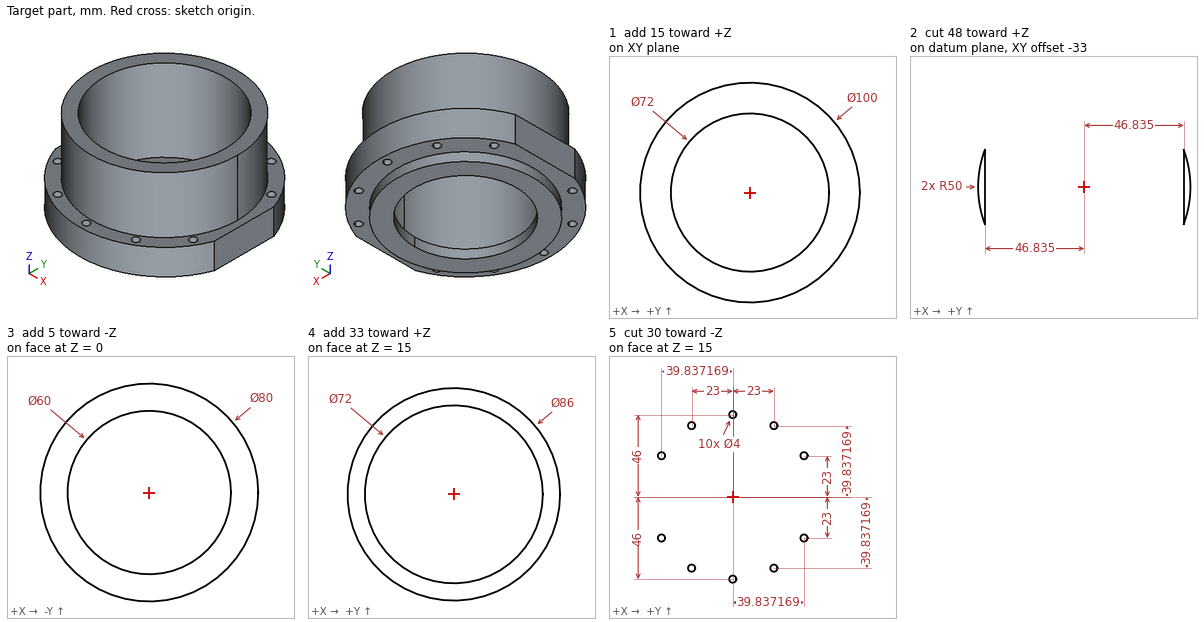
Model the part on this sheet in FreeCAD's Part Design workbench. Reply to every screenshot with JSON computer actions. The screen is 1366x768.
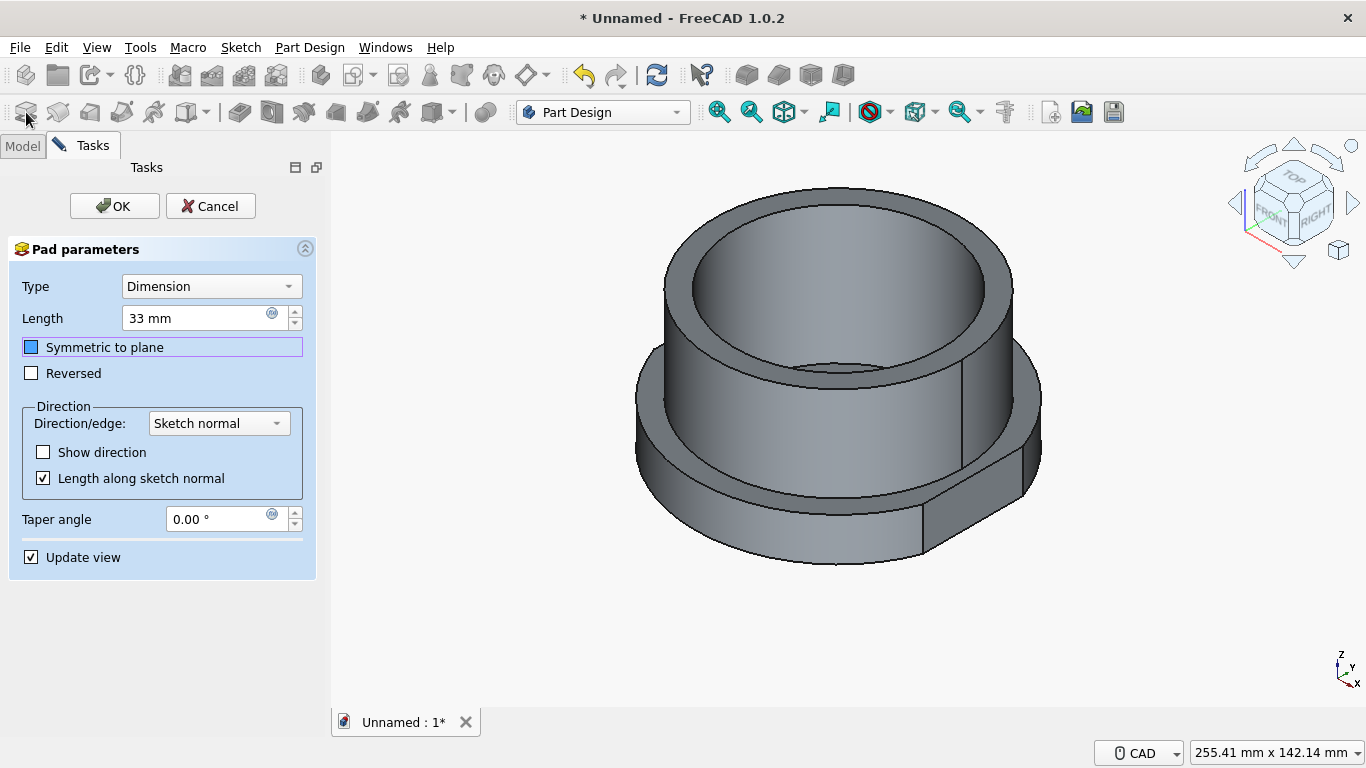
{"action": "left_click", "coordinate": [115, 206]}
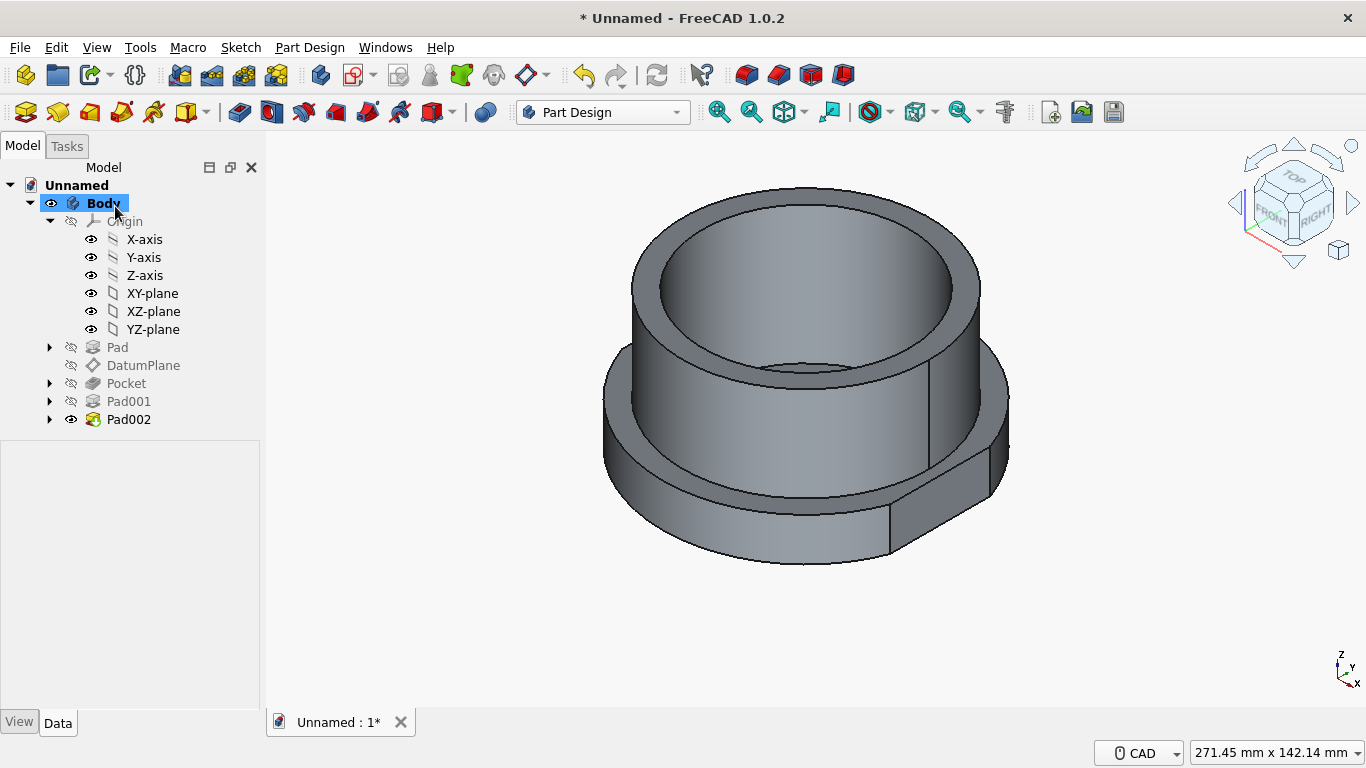
{"action": "left_click", "coordinate": [720, 112]}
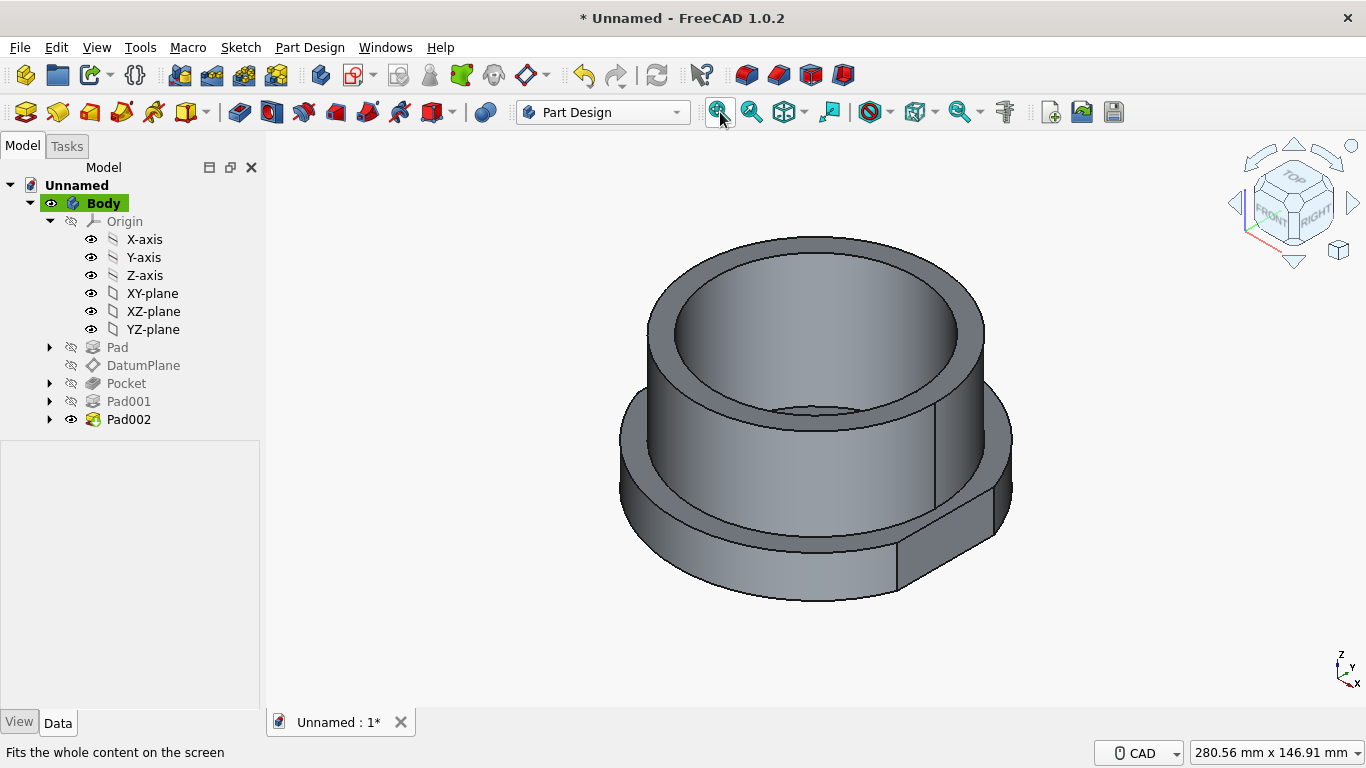
{"action": "left_click", "coordinate": [660, 486]}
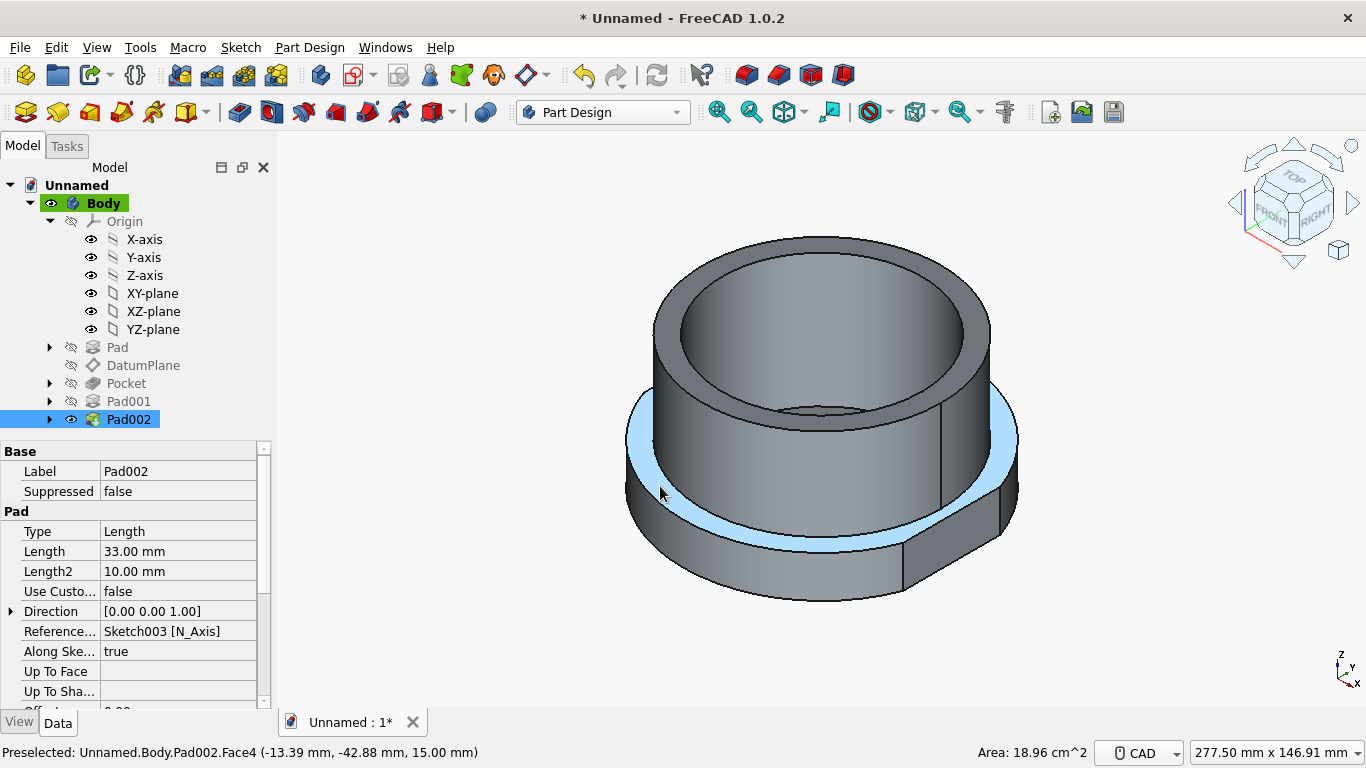
{"action": "left_click", "coordinate": [354, 76]}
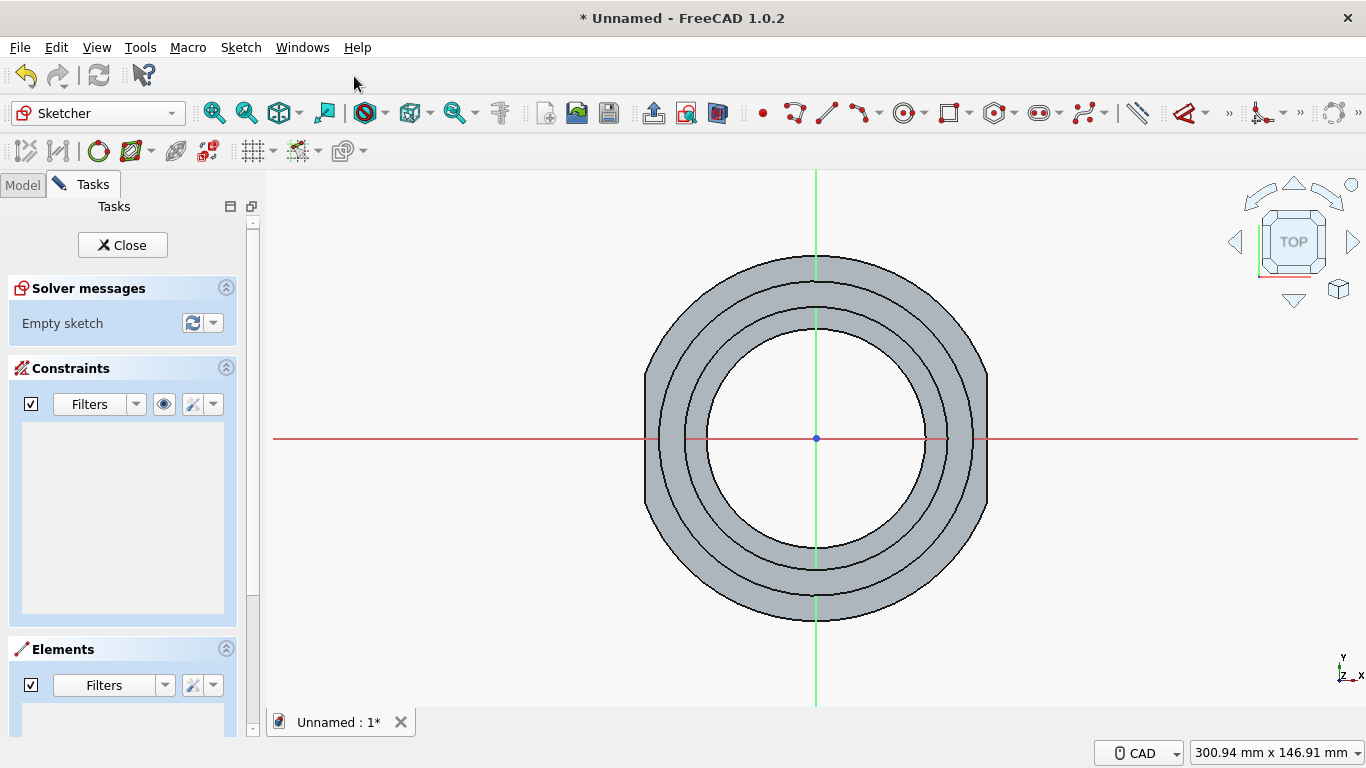
{"action": "left_click", "coordinate": [718, 114]}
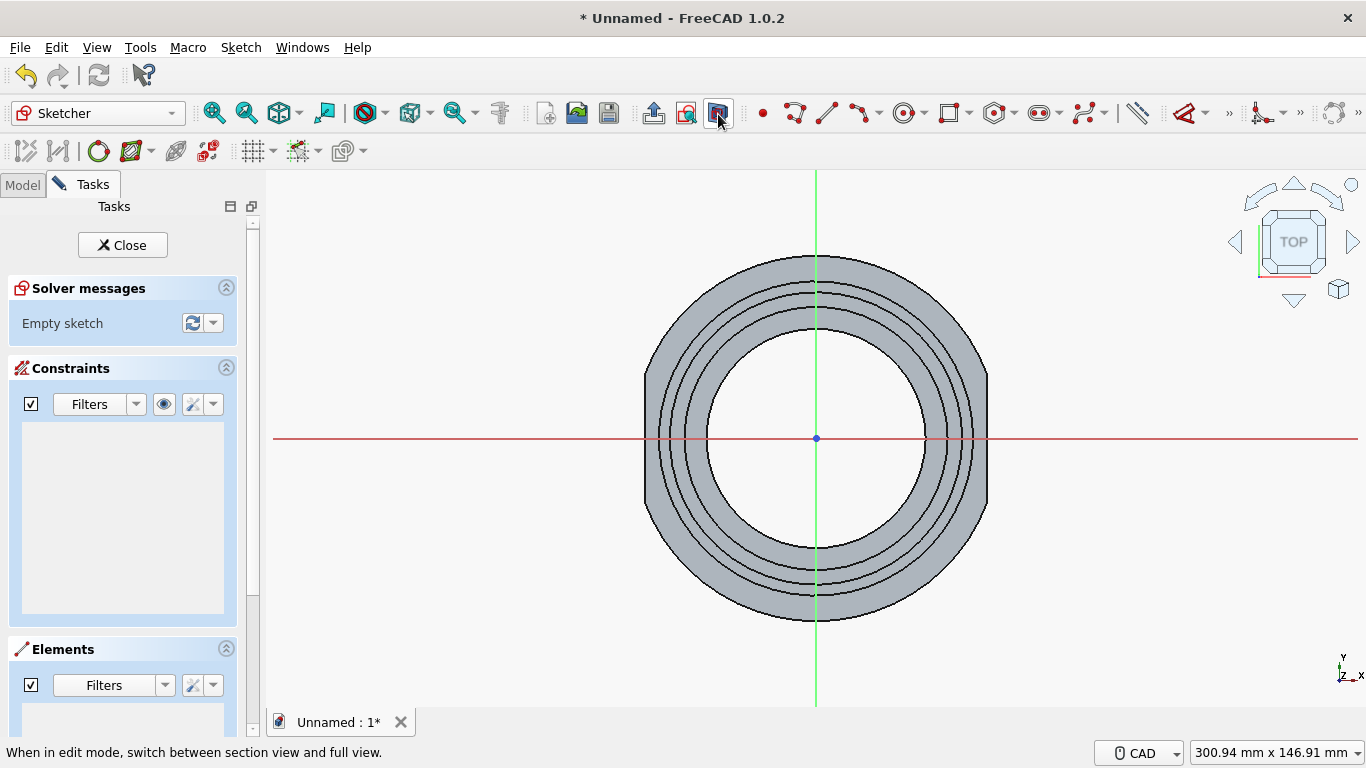
{"action": "left_click", "coordinate": [904, 114]}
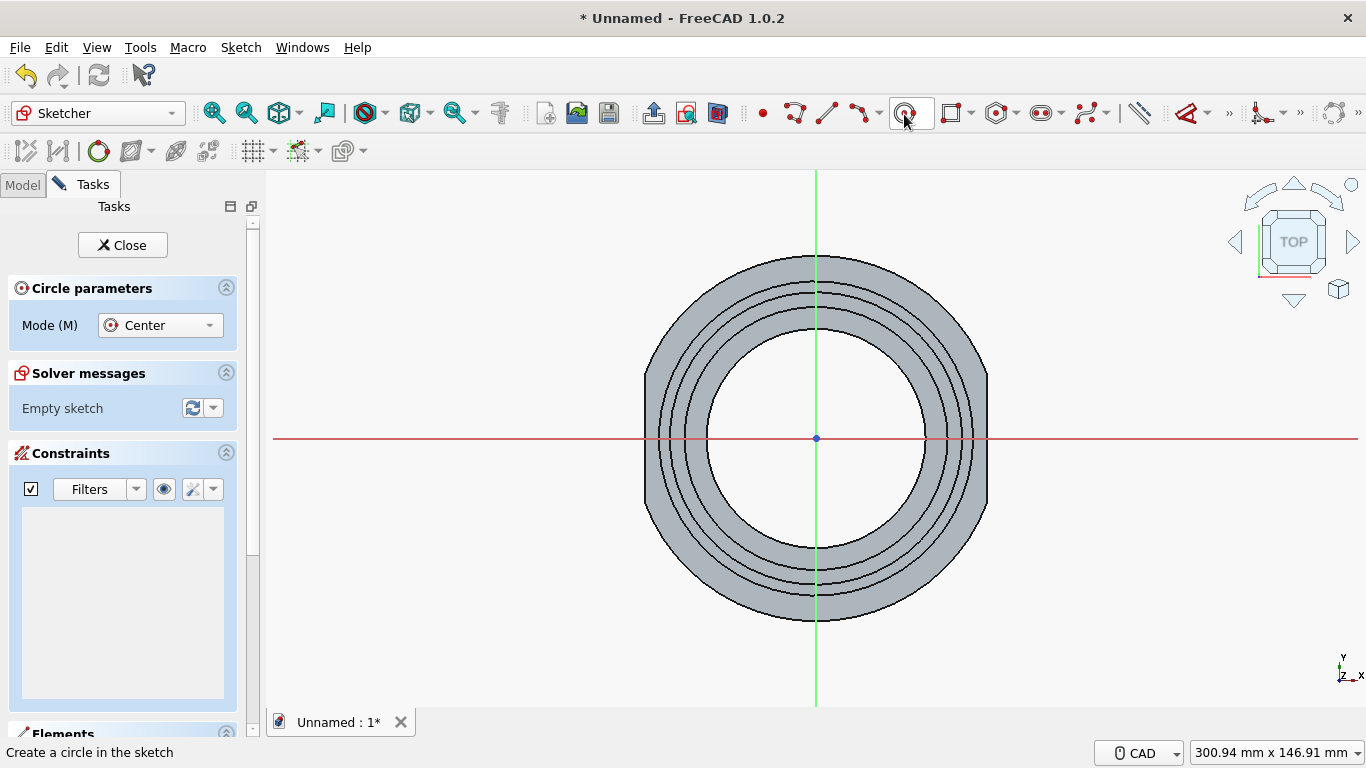
{"action": "scroll", "coordinate": [816, 270], "scroll_direction": "up", "scroll_amount": 6}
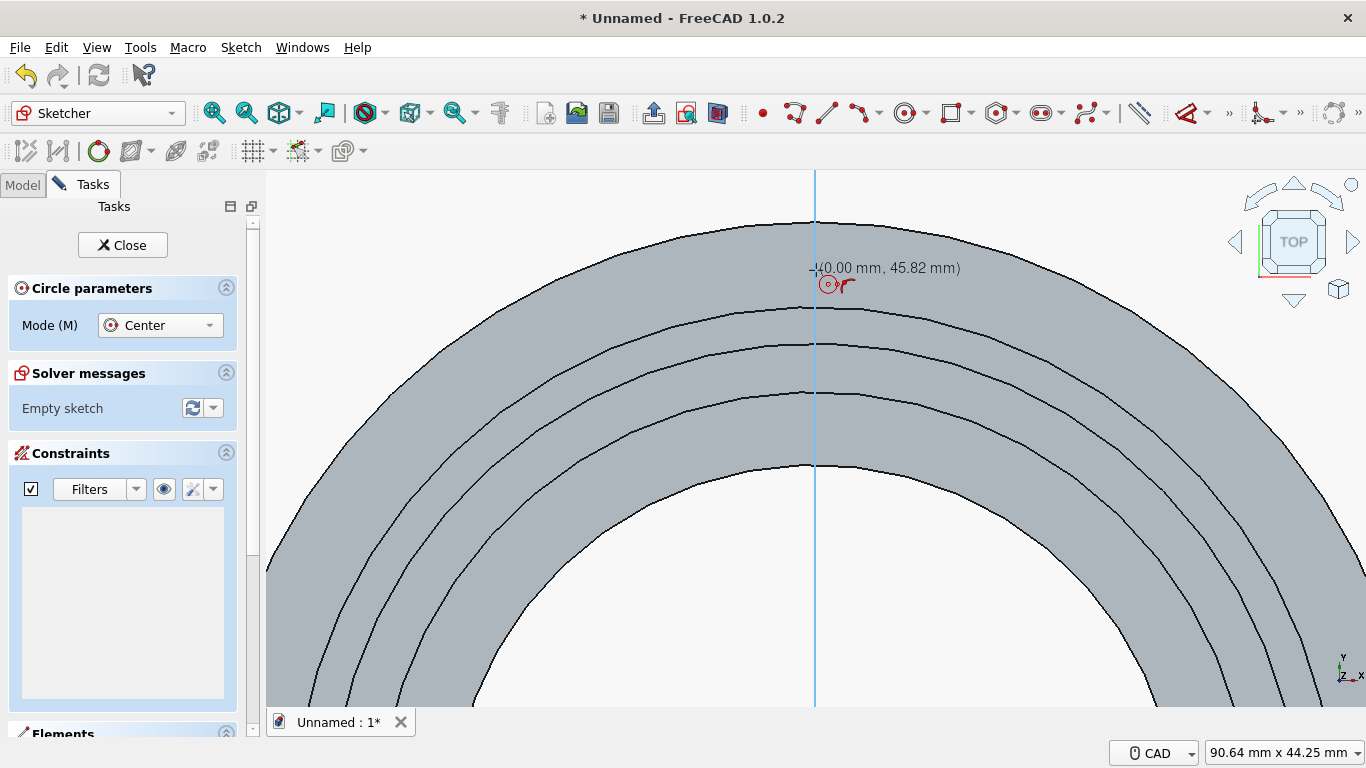
{"action": "left_click", "coordinate": [815, 271]}
{"action": "mouse_move", "coordinate": [832, 254]}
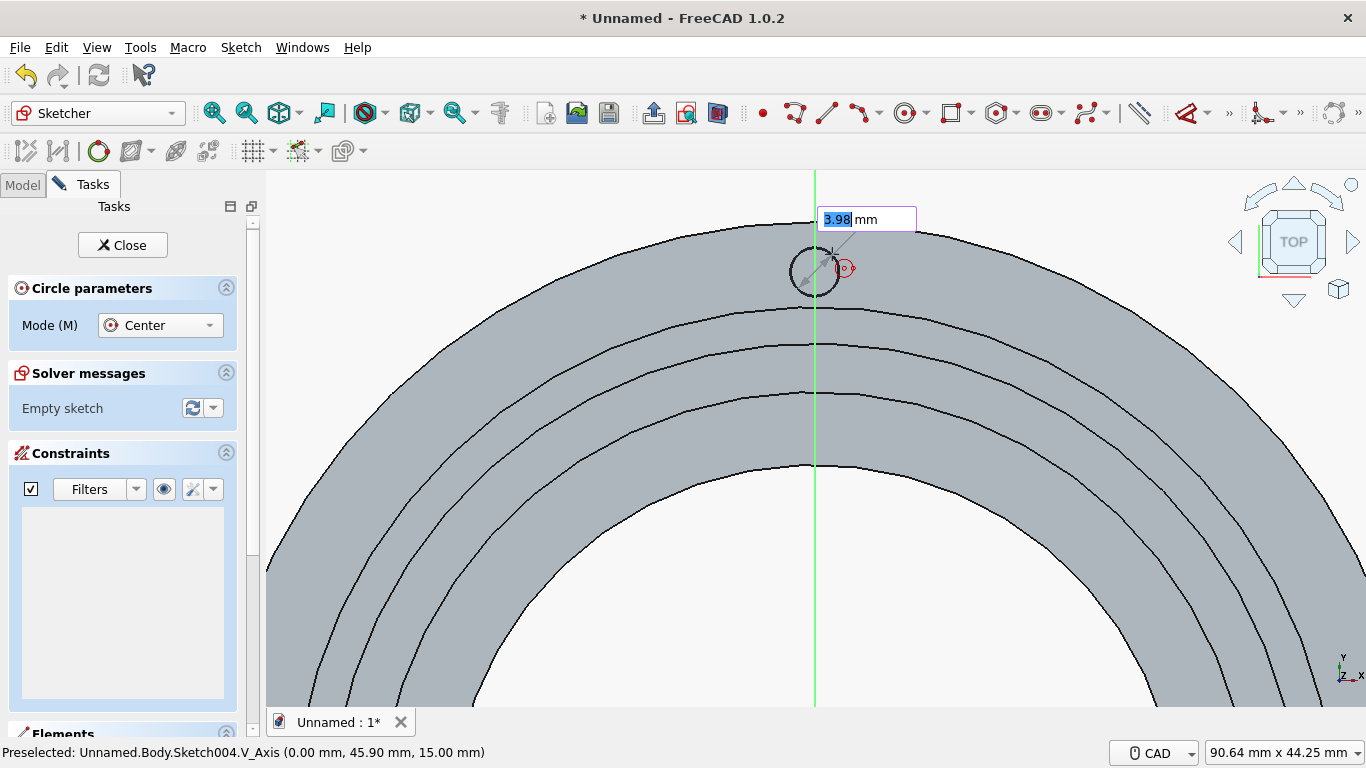
{"action": "type", "text": "4"}
{"action": "key", "text": "Return"}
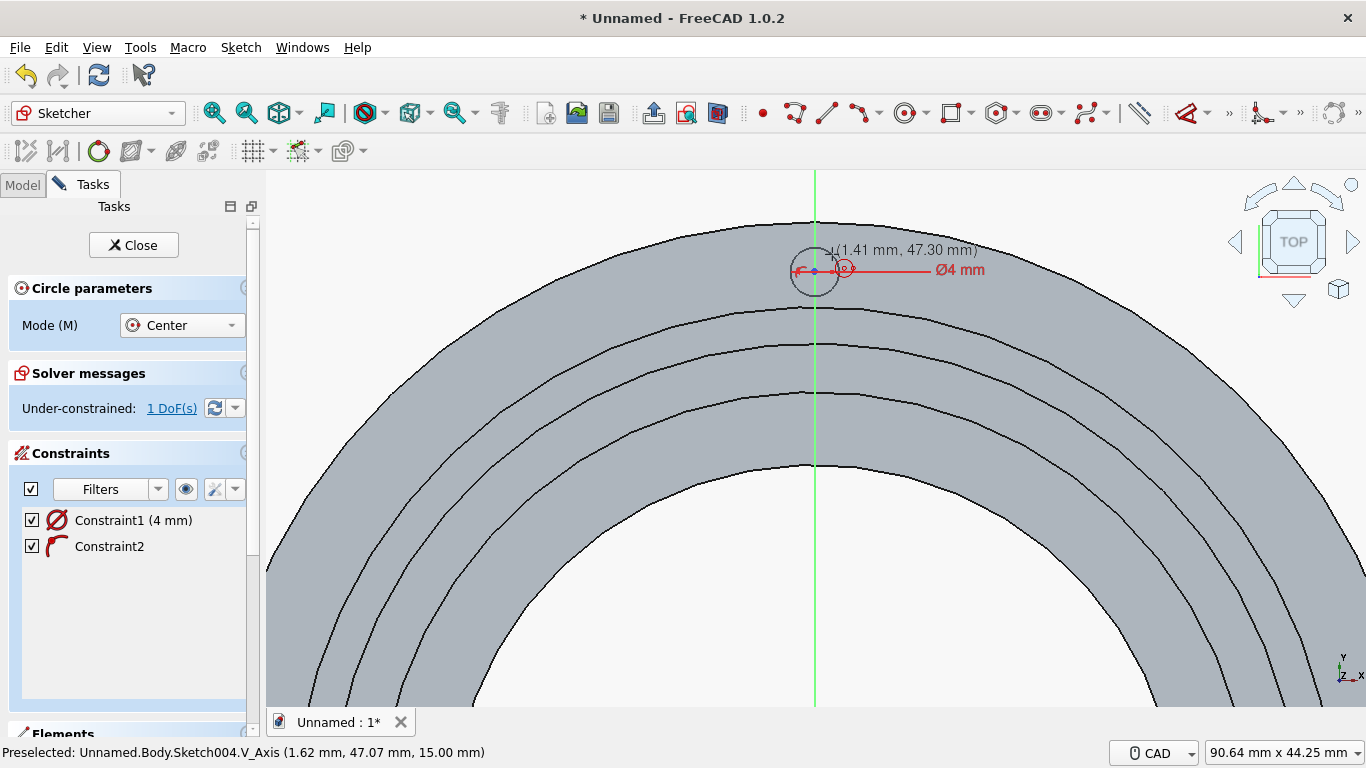
{"action": "scroll", "coordinate": [718, 270], "scroll_direction": "down", "scroll_amount": 6}